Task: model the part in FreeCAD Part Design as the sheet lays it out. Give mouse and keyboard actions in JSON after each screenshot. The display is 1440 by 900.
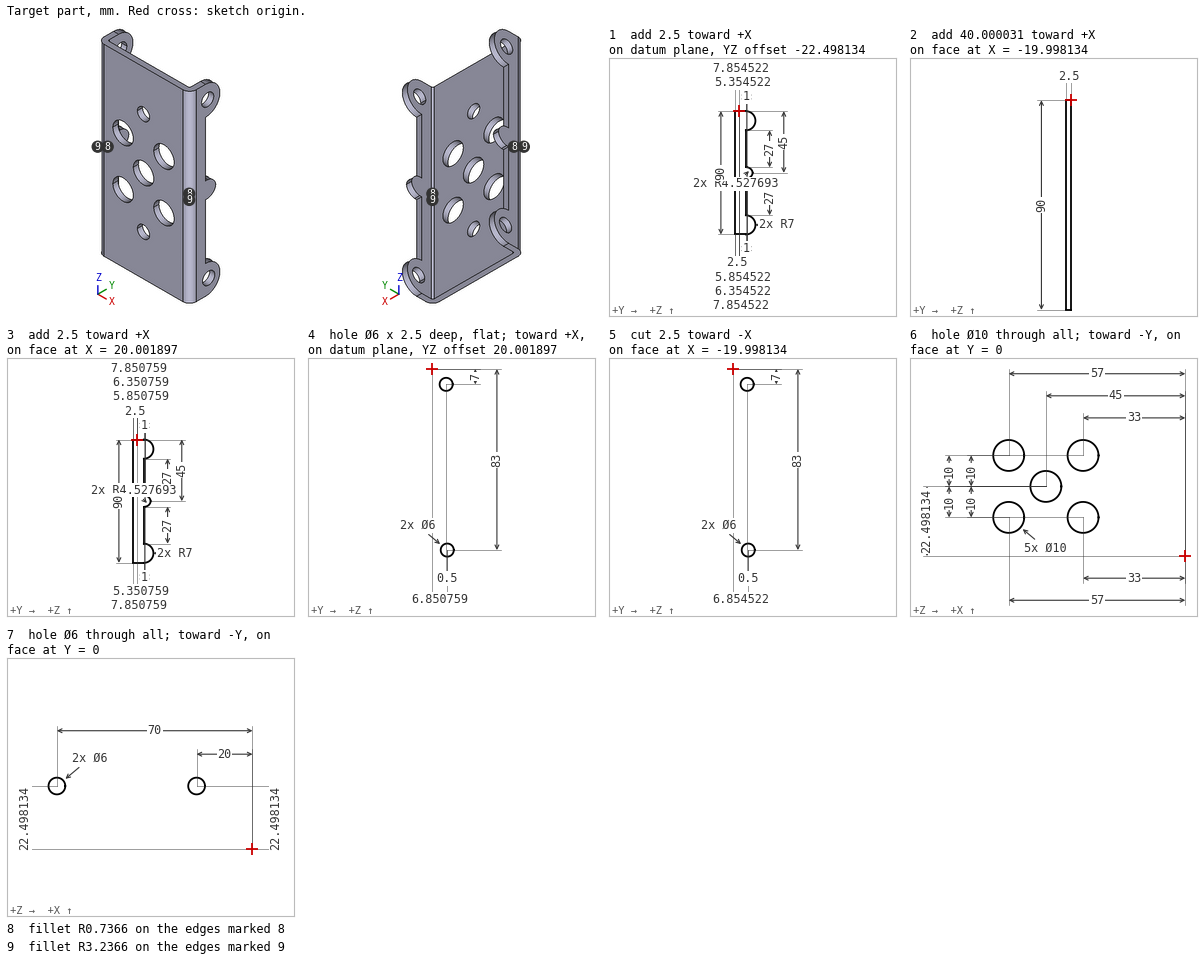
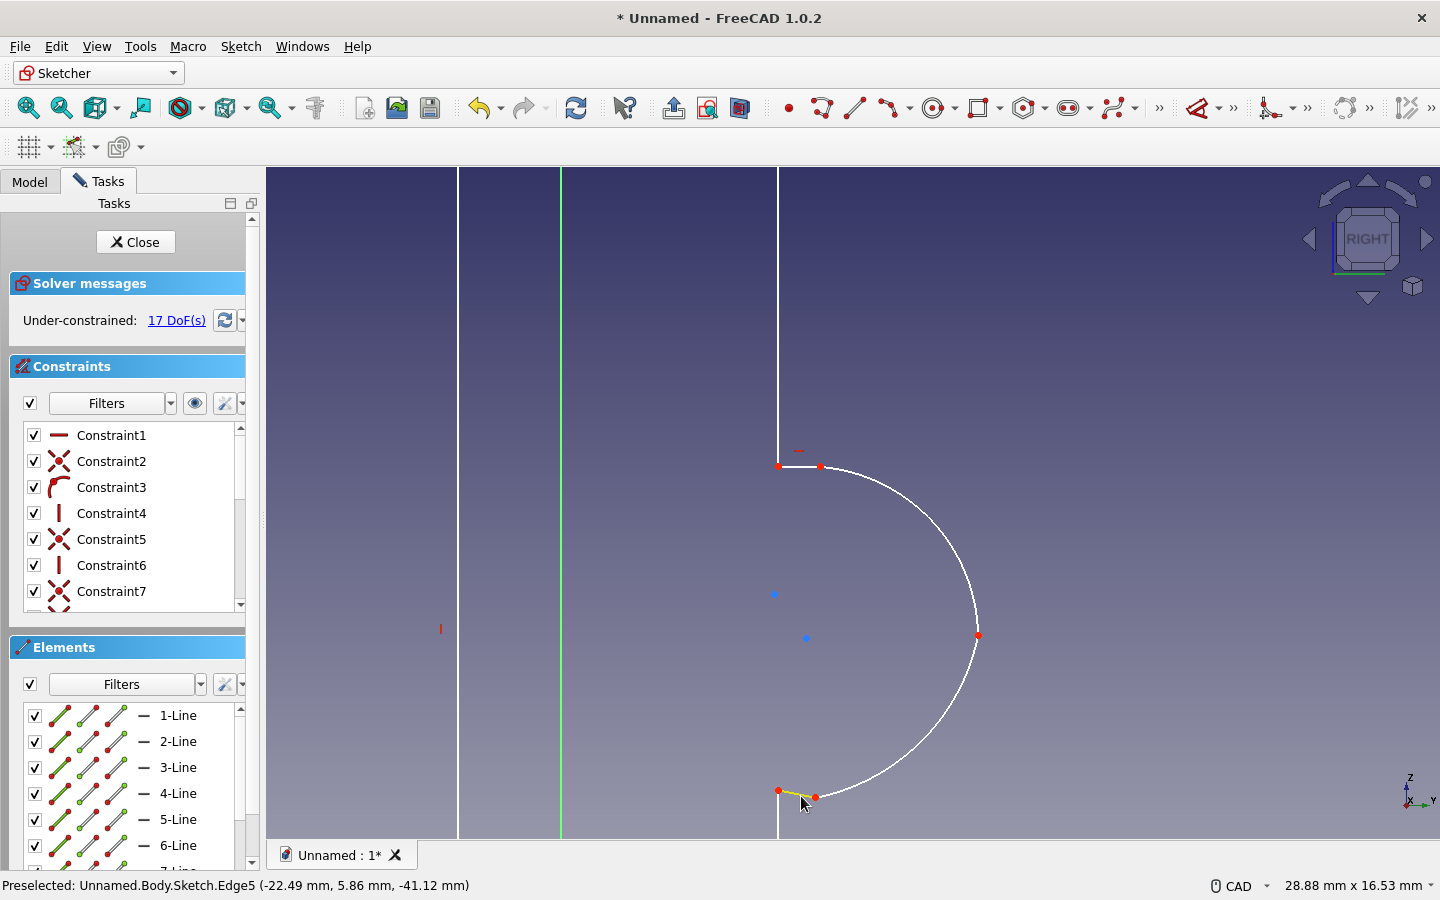
{"action": "left_click", "coordinate": [801, 795]}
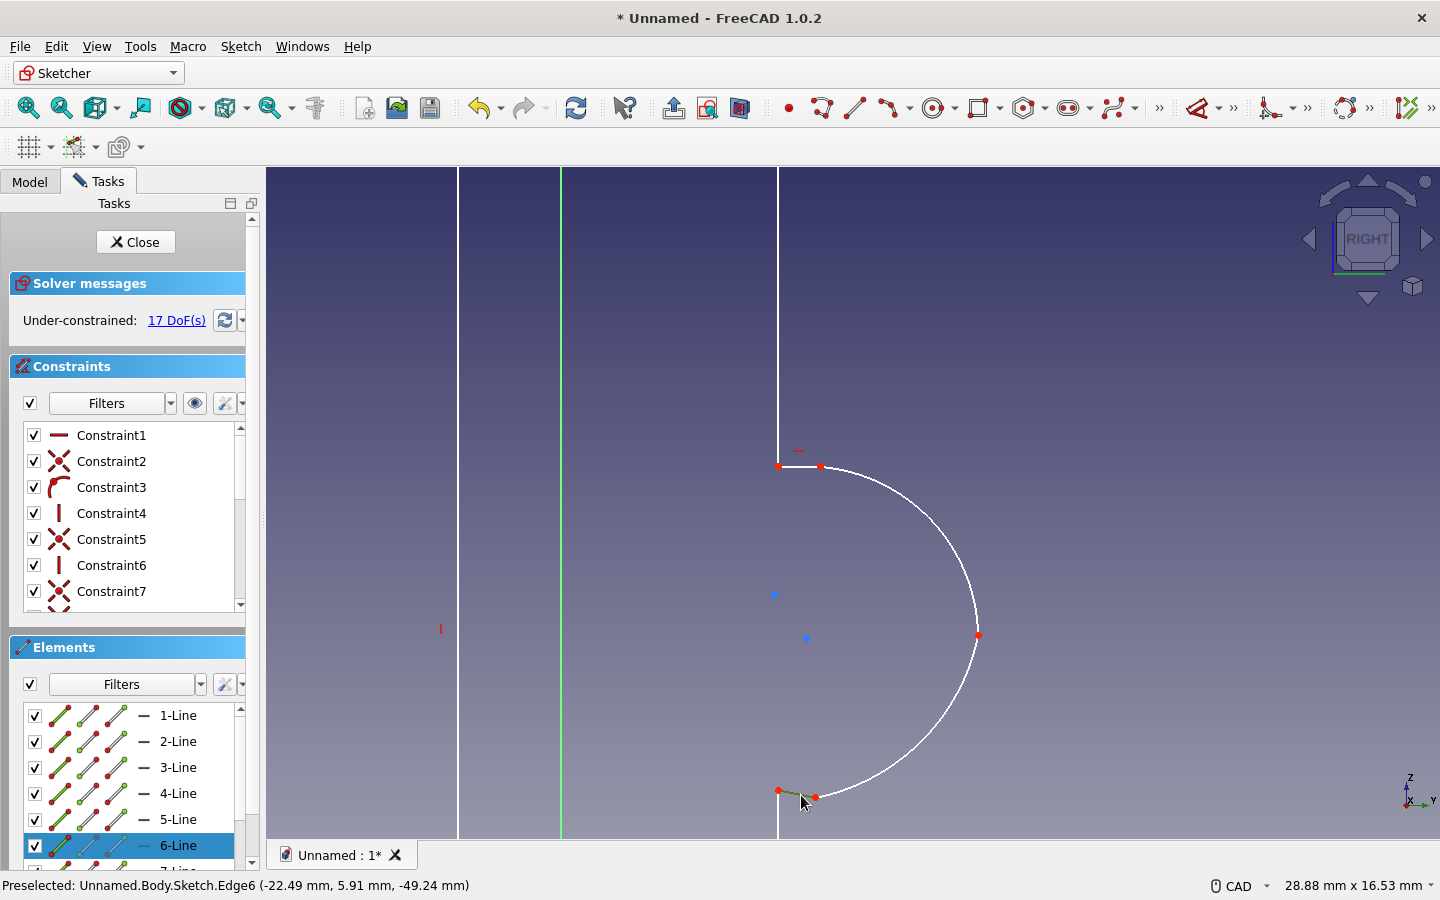
{"action": "key", "text": "h"}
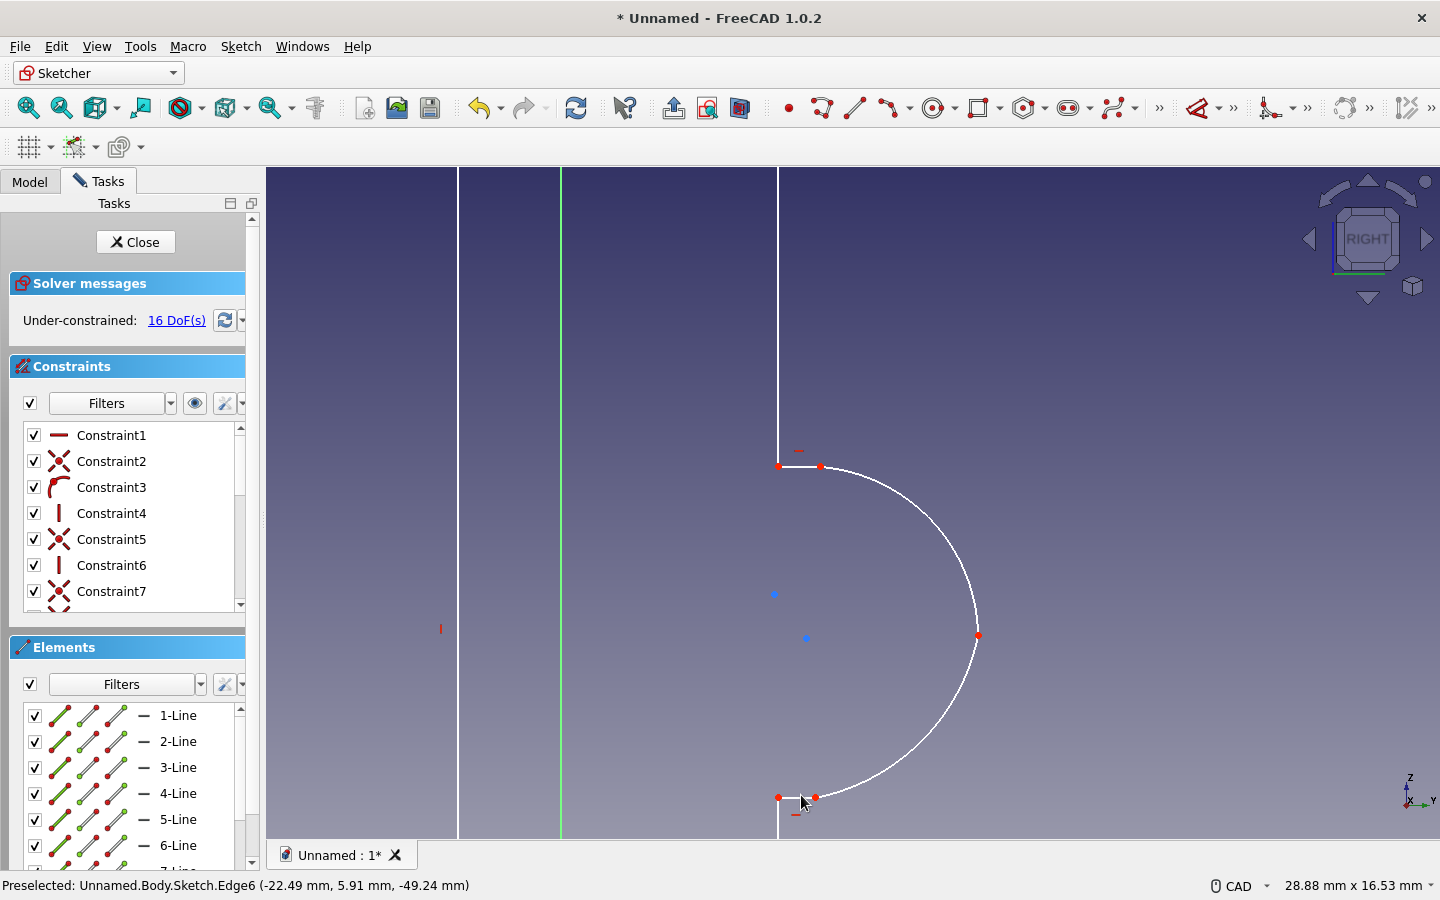
{"action": "scroll", "coordinate": [787, 488], "scroll_direction": "down", "scroll_amount": 11}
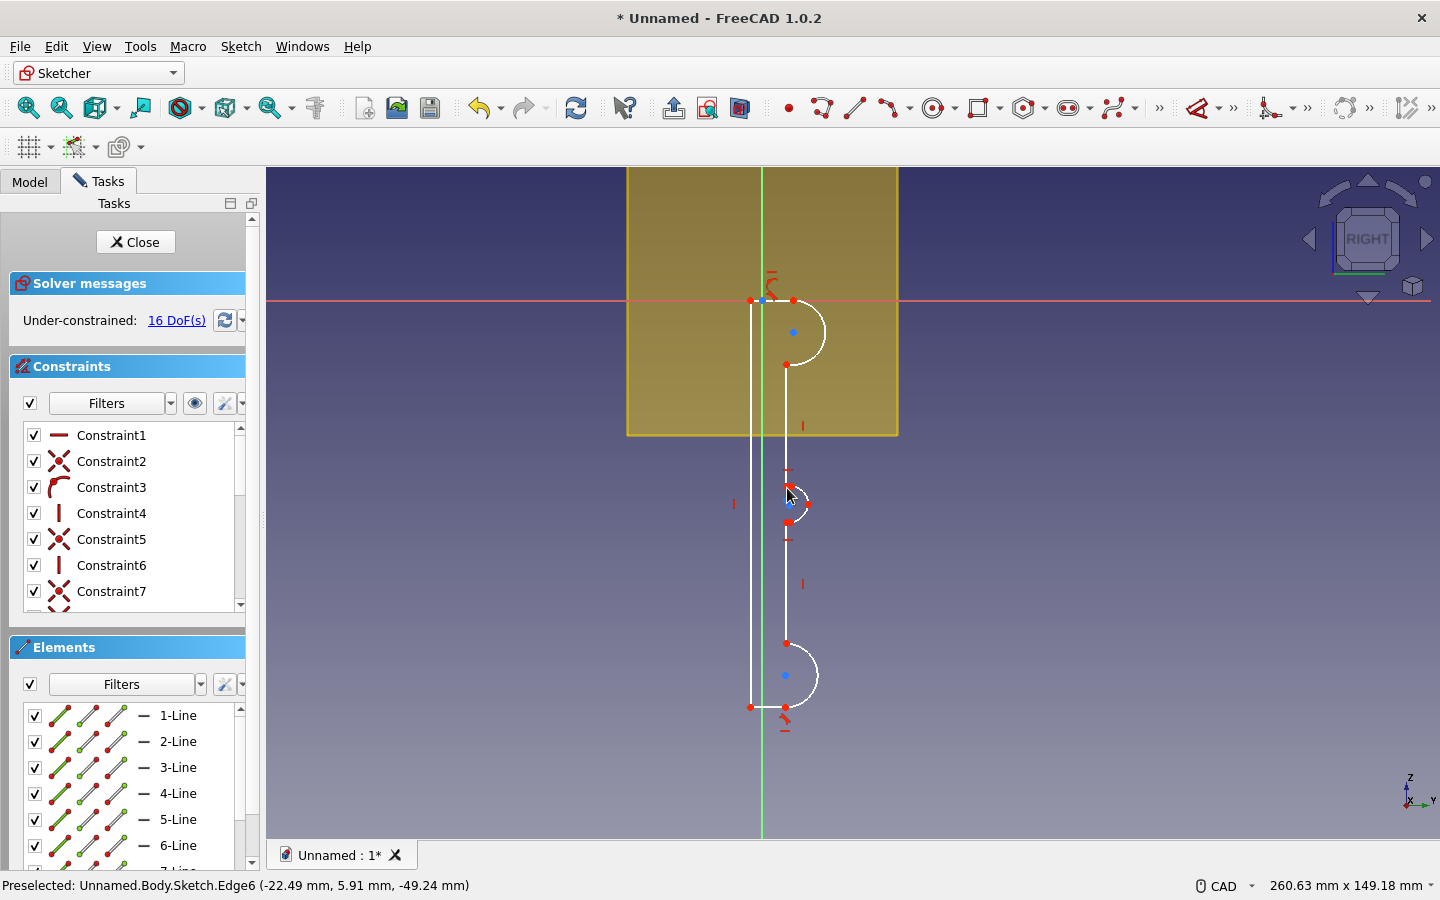
{"action": "scroll", "coordinate": [807, 497], "scroll_direction": "up", "scroll_amount": 3}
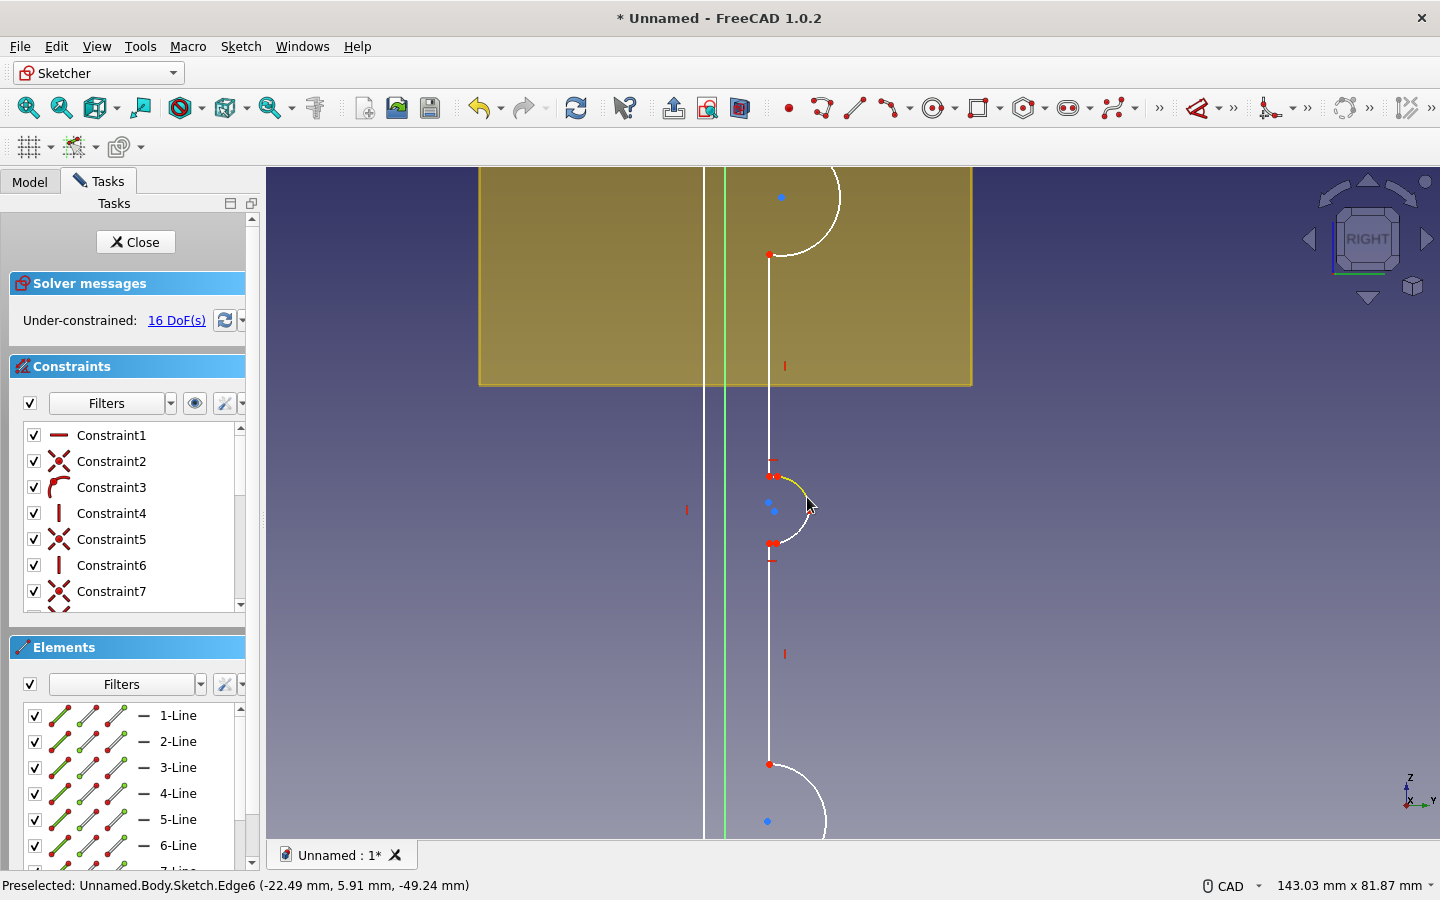
{"action": "left_click", "coordinate": [806, 496]}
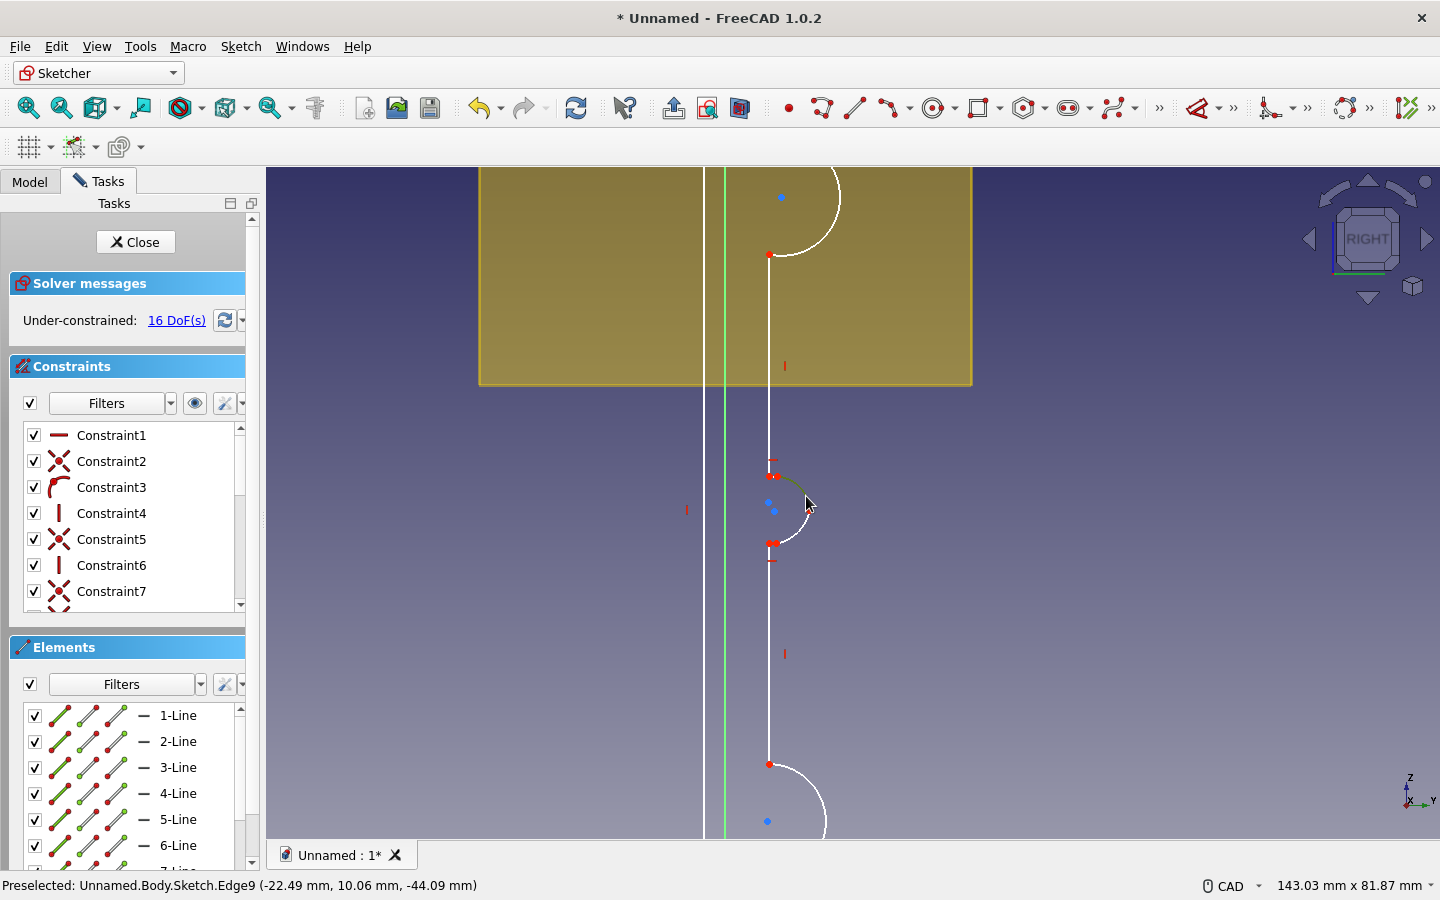
{"action": "left_click", "coordinate": [790, 538]}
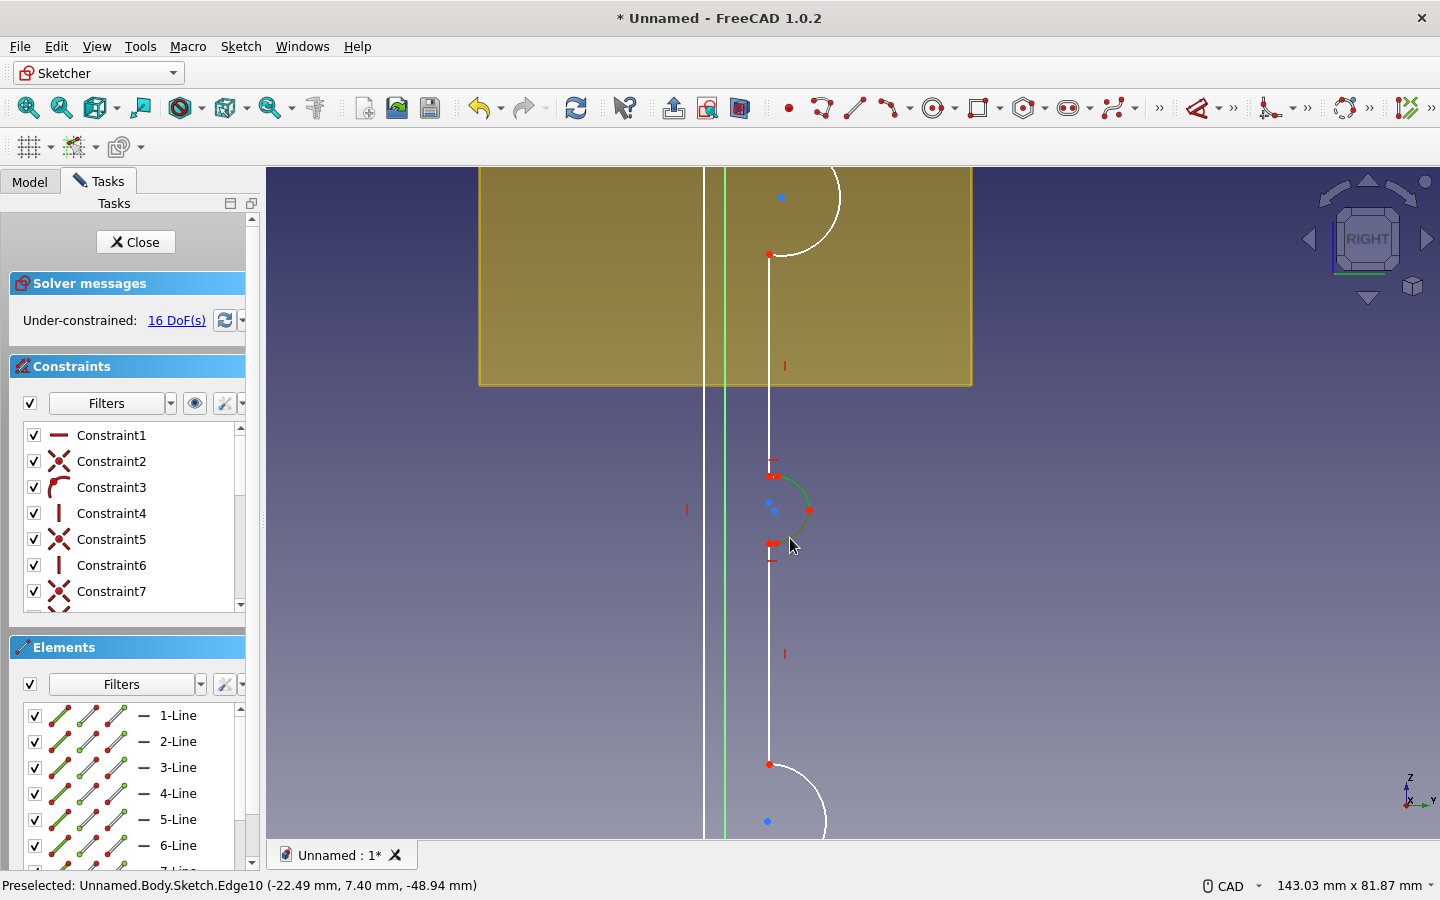
{"action": "key", "text": "e"}